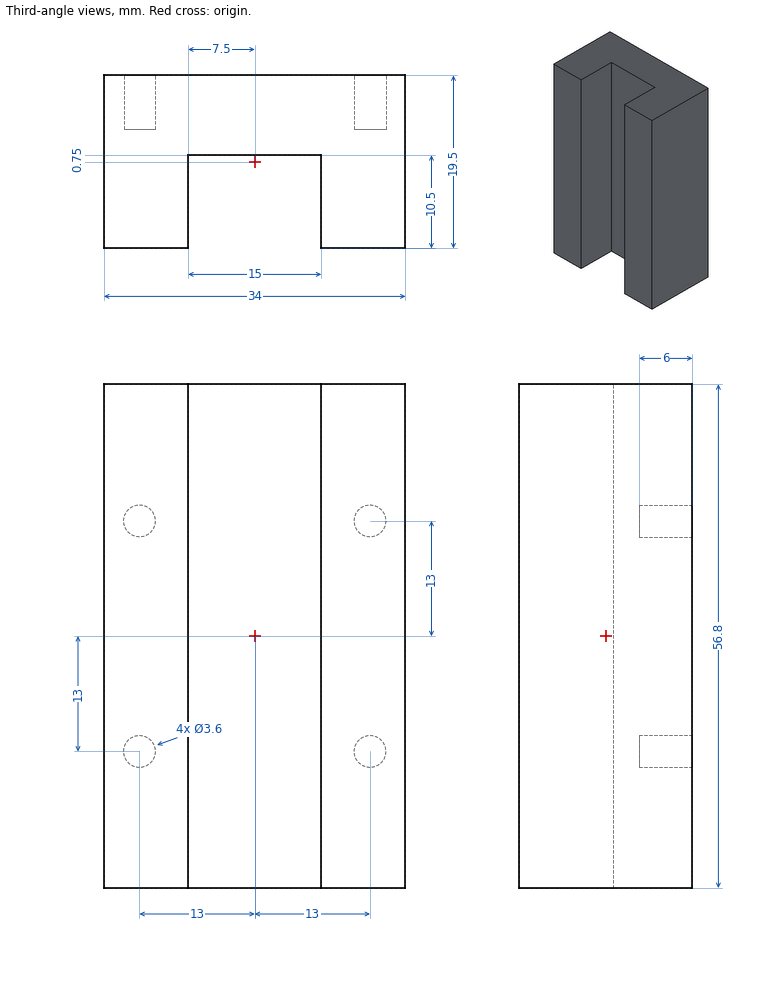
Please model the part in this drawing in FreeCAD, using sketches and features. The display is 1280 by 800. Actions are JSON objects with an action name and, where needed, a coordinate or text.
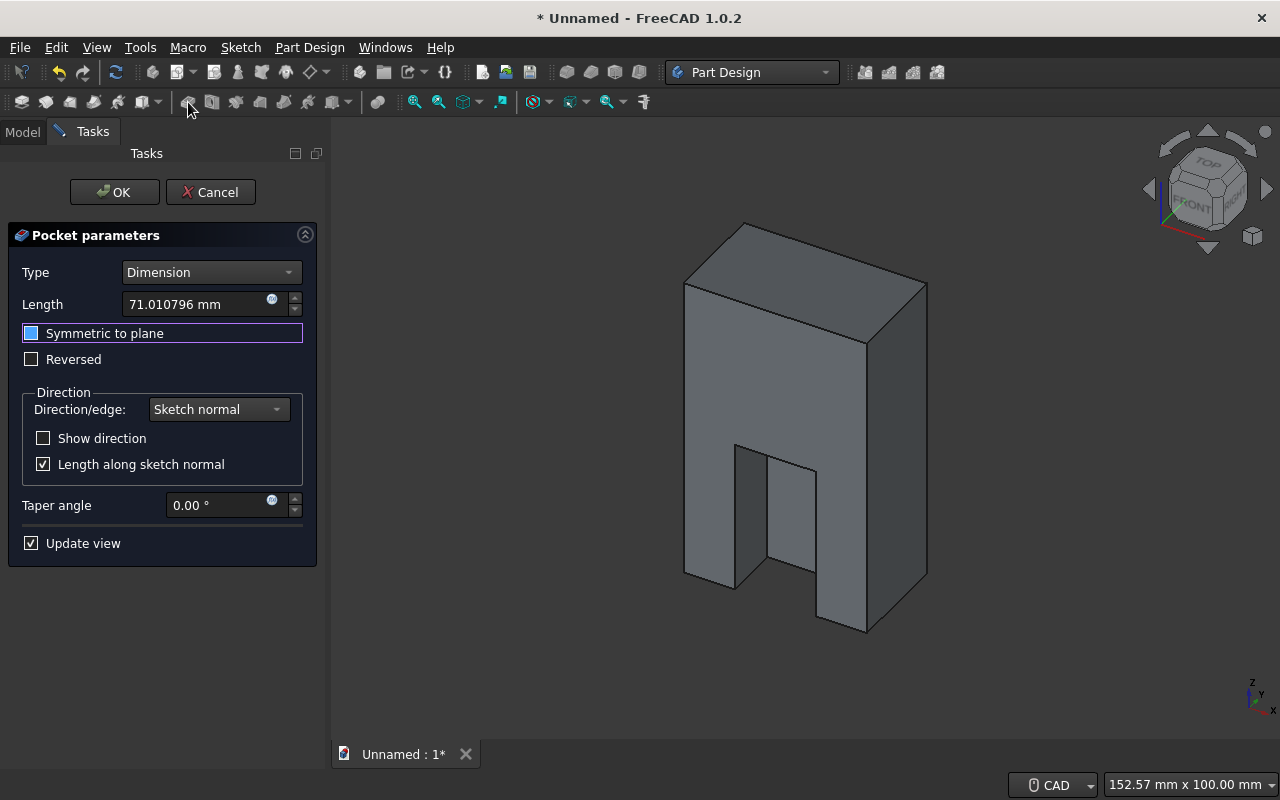
{"action": "left_click", "coordinate": [30, 333]}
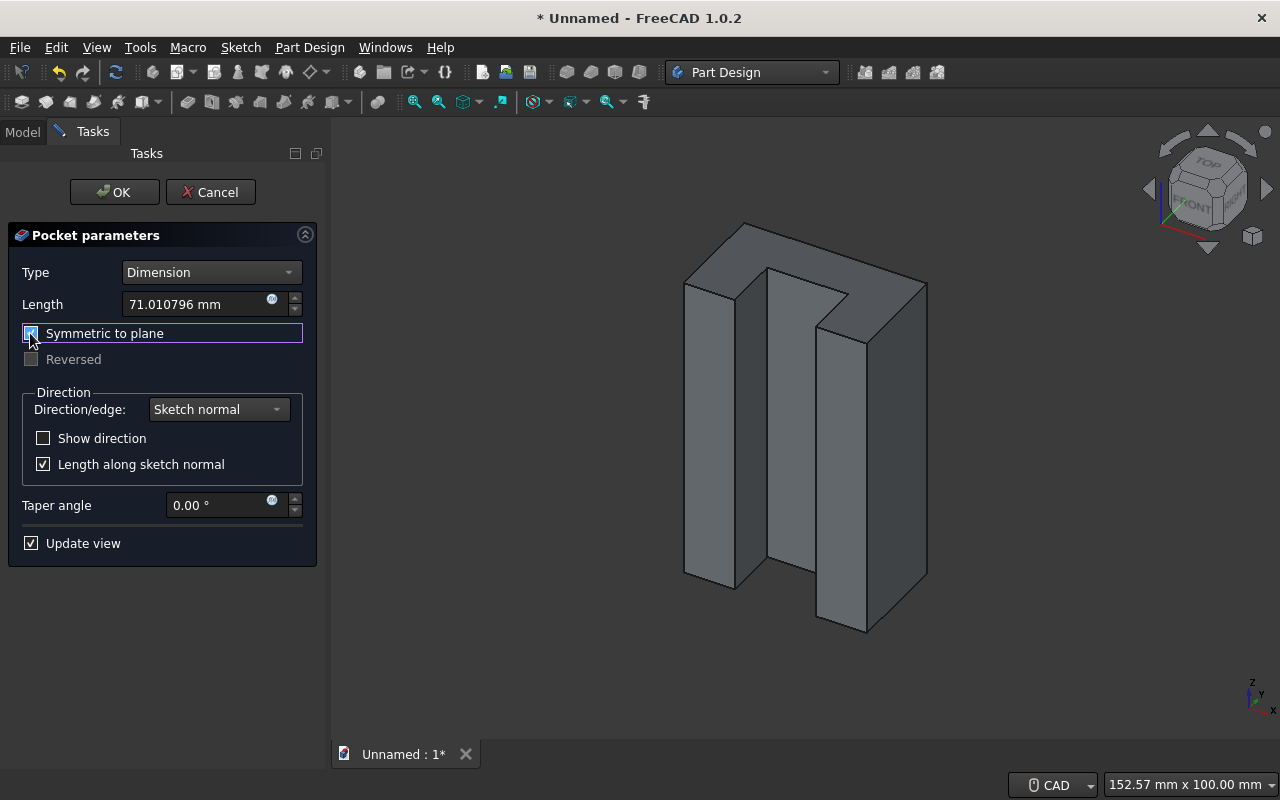
{"action": "left_click", "coordinate": [115, 192]}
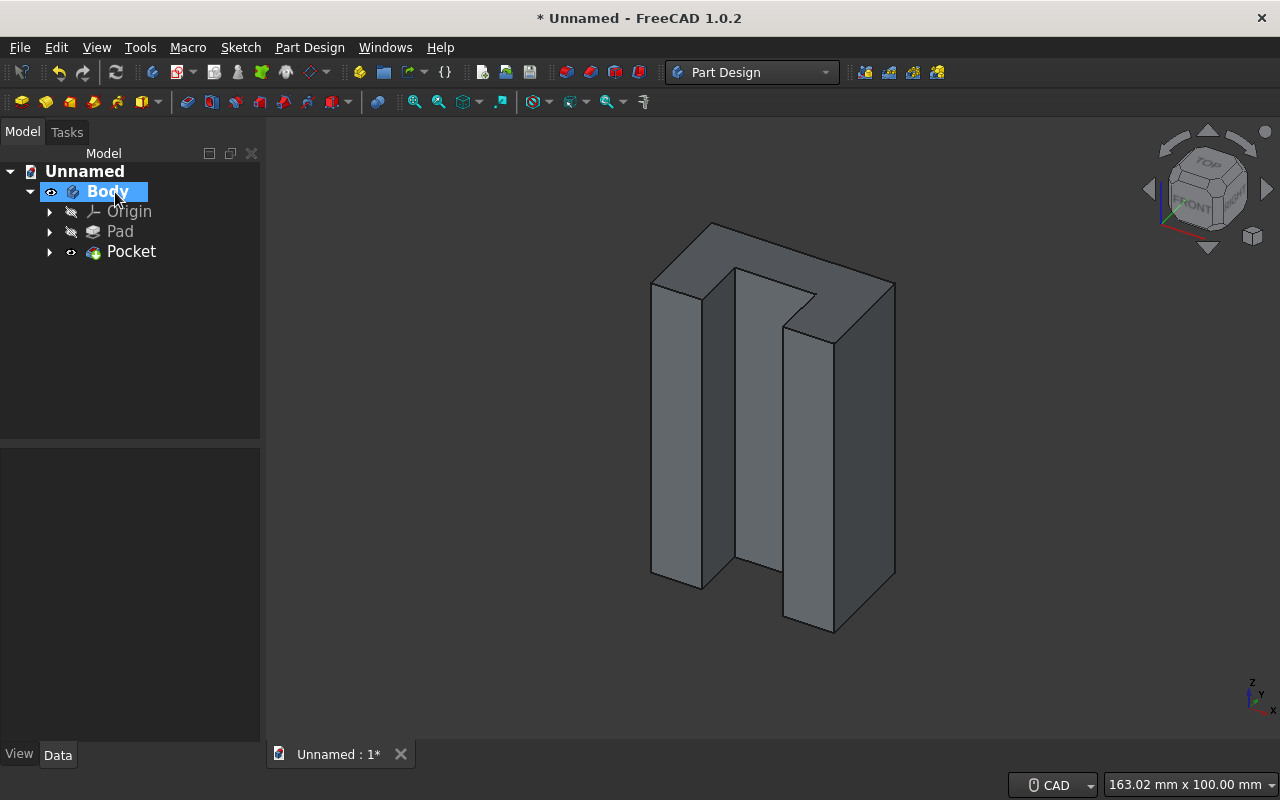
{"action": "key", "text": "4"}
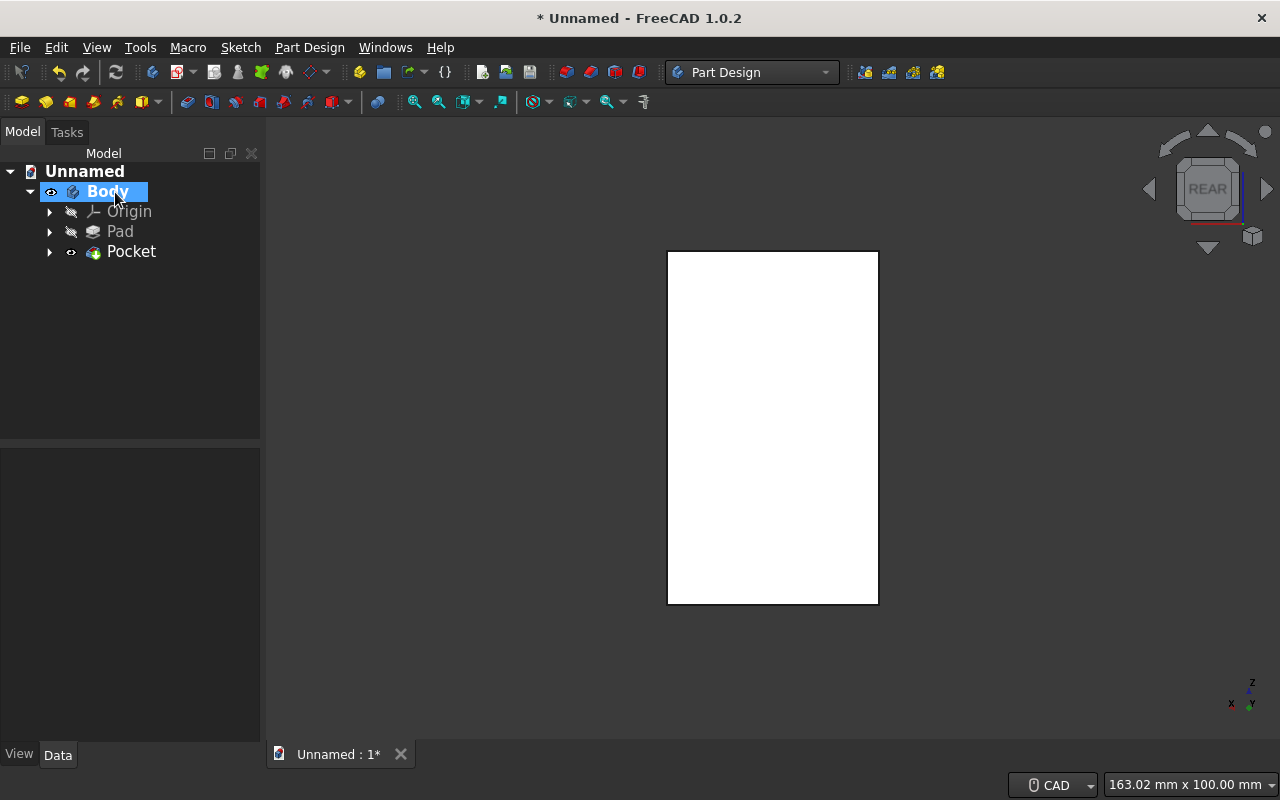
{"action": "left_click", "coordinate": [773, 377]}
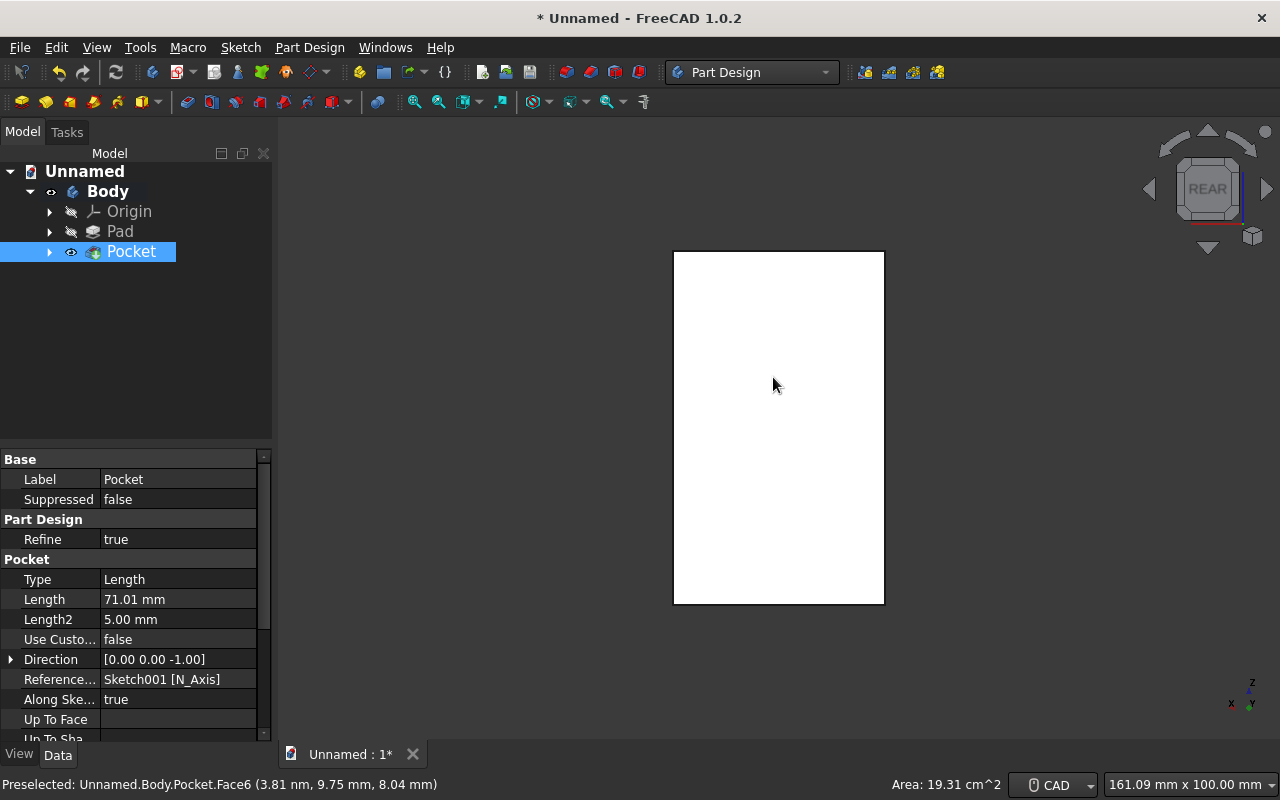
{"action": "left_click", "coordinate": [178, 72]}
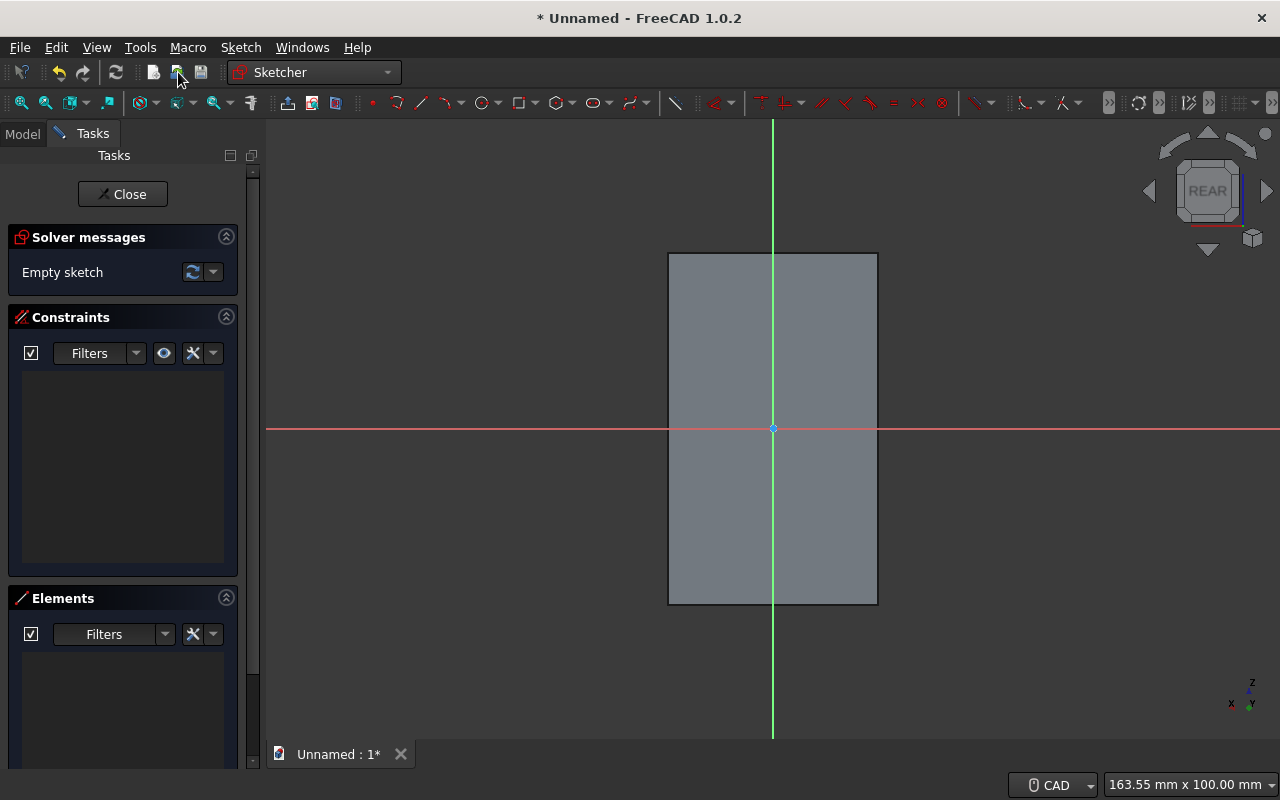
{"action": "scroll", "coordinate": [829, 429], "scroll_direction": "up", "scroll_amount": 4}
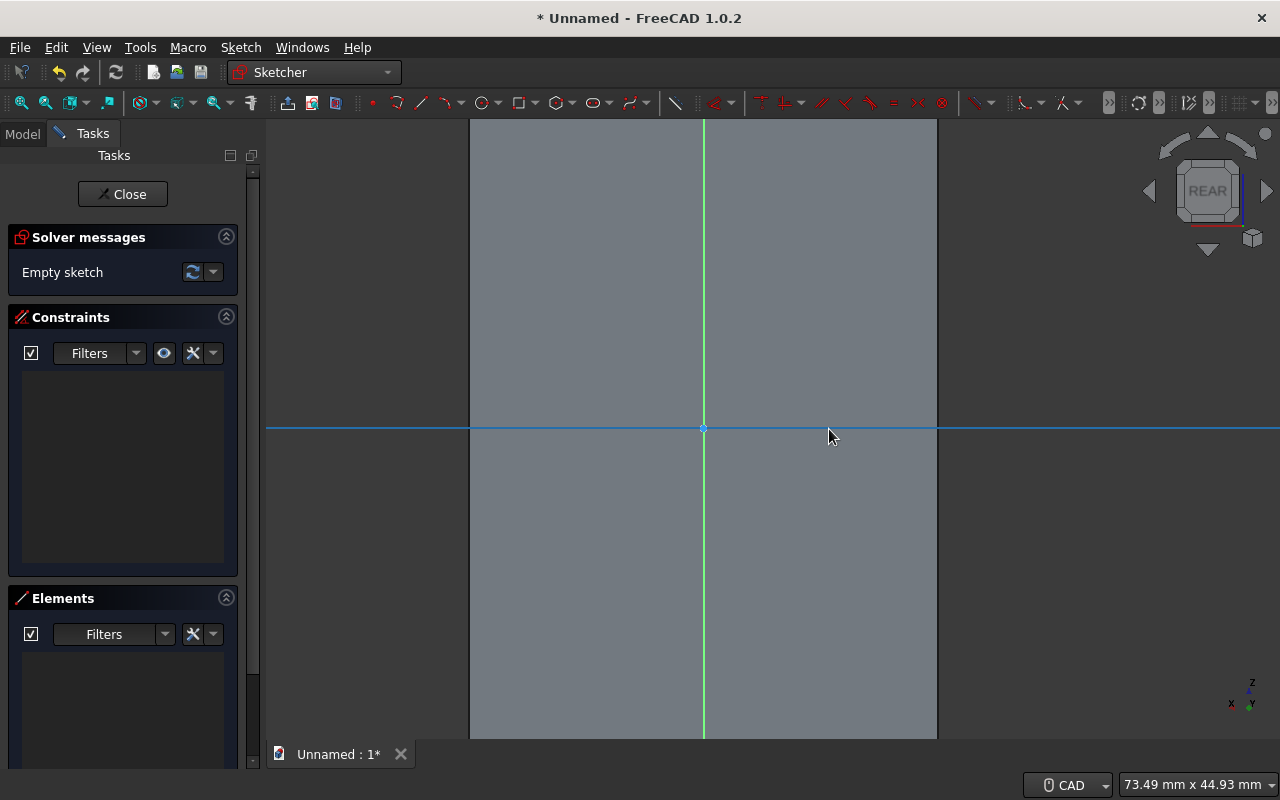
{"action": "left_click", "coordinate": [482, 104]}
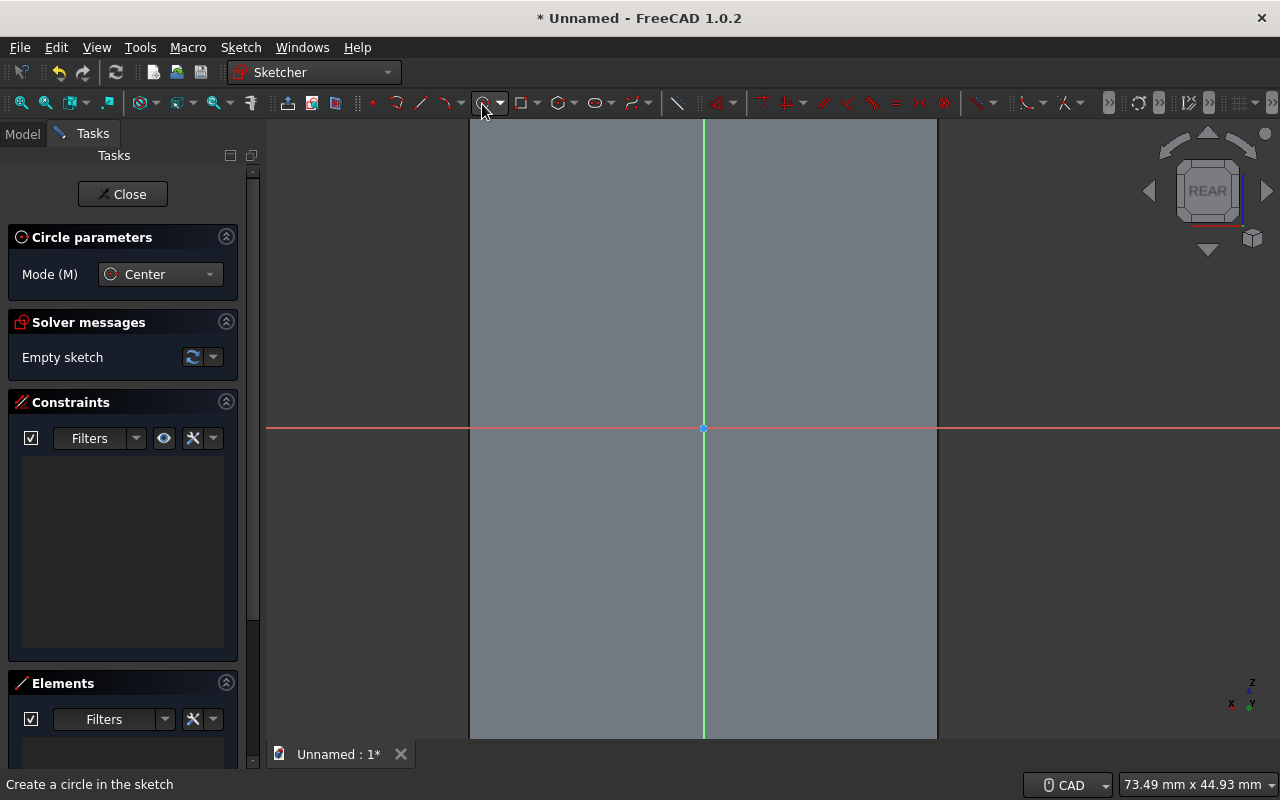
{"action": "left_click", "coordinate": [883, 608]}
{"action": "mouse_move", "coordinate": [901, 590]}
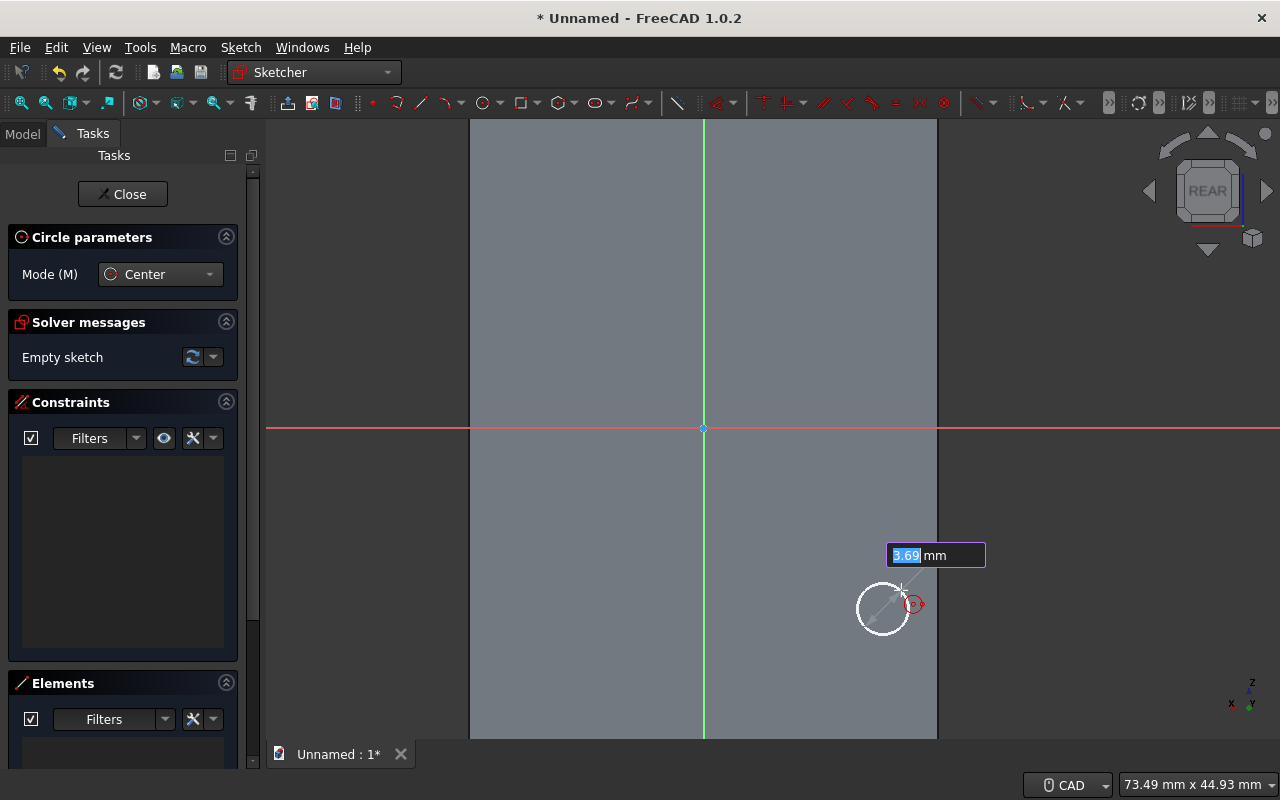
{"action": "type", "text": "3.6"}
{"action": "key", "text": "Return"}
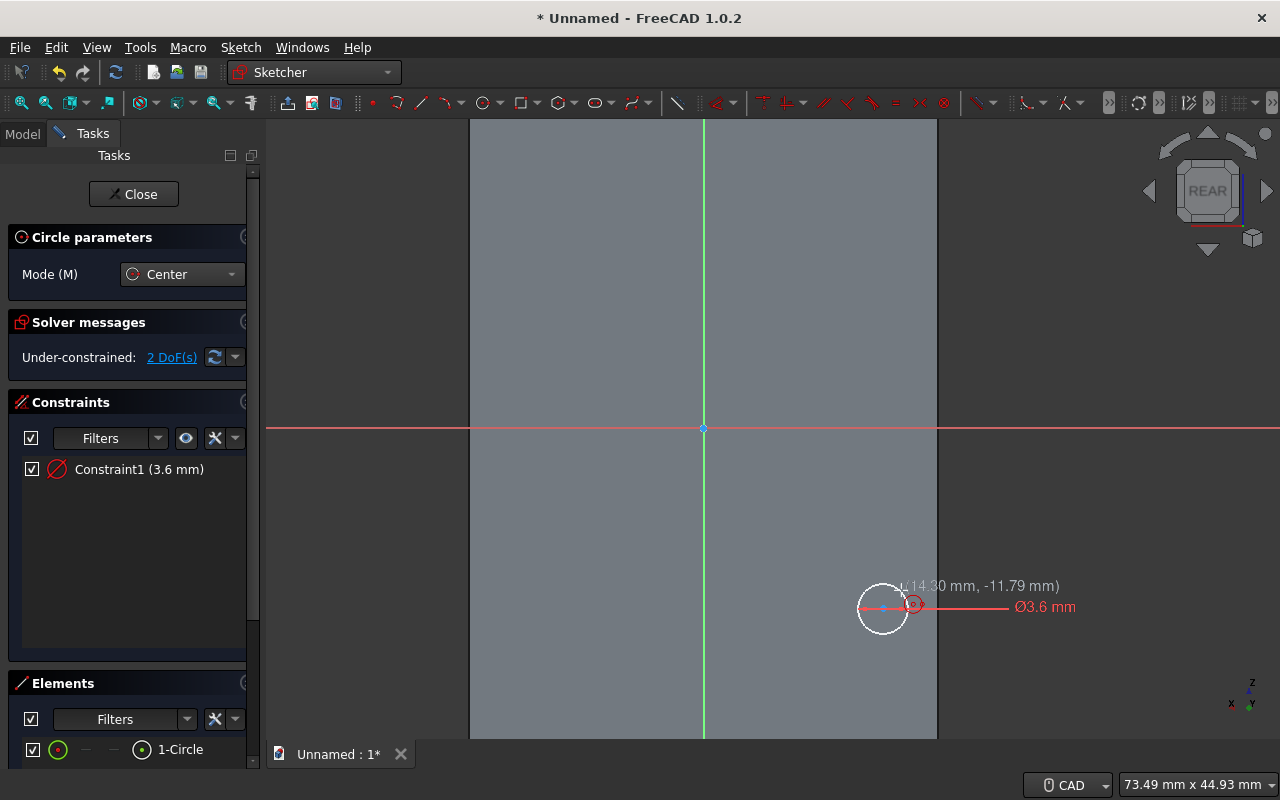
{"action": "left_click", "coordinate": [524, 608]}
{"action": "mouse_move", "coordinate": [542, 590]}